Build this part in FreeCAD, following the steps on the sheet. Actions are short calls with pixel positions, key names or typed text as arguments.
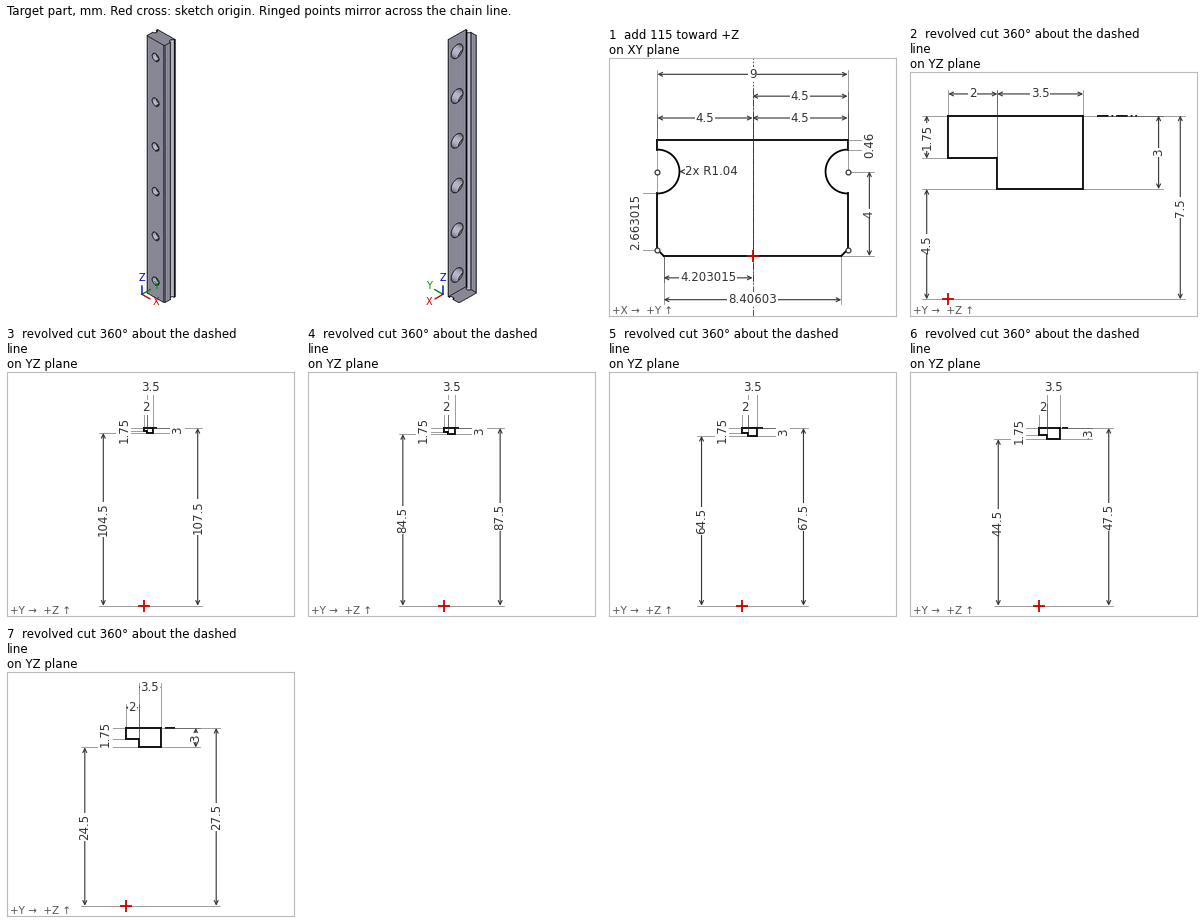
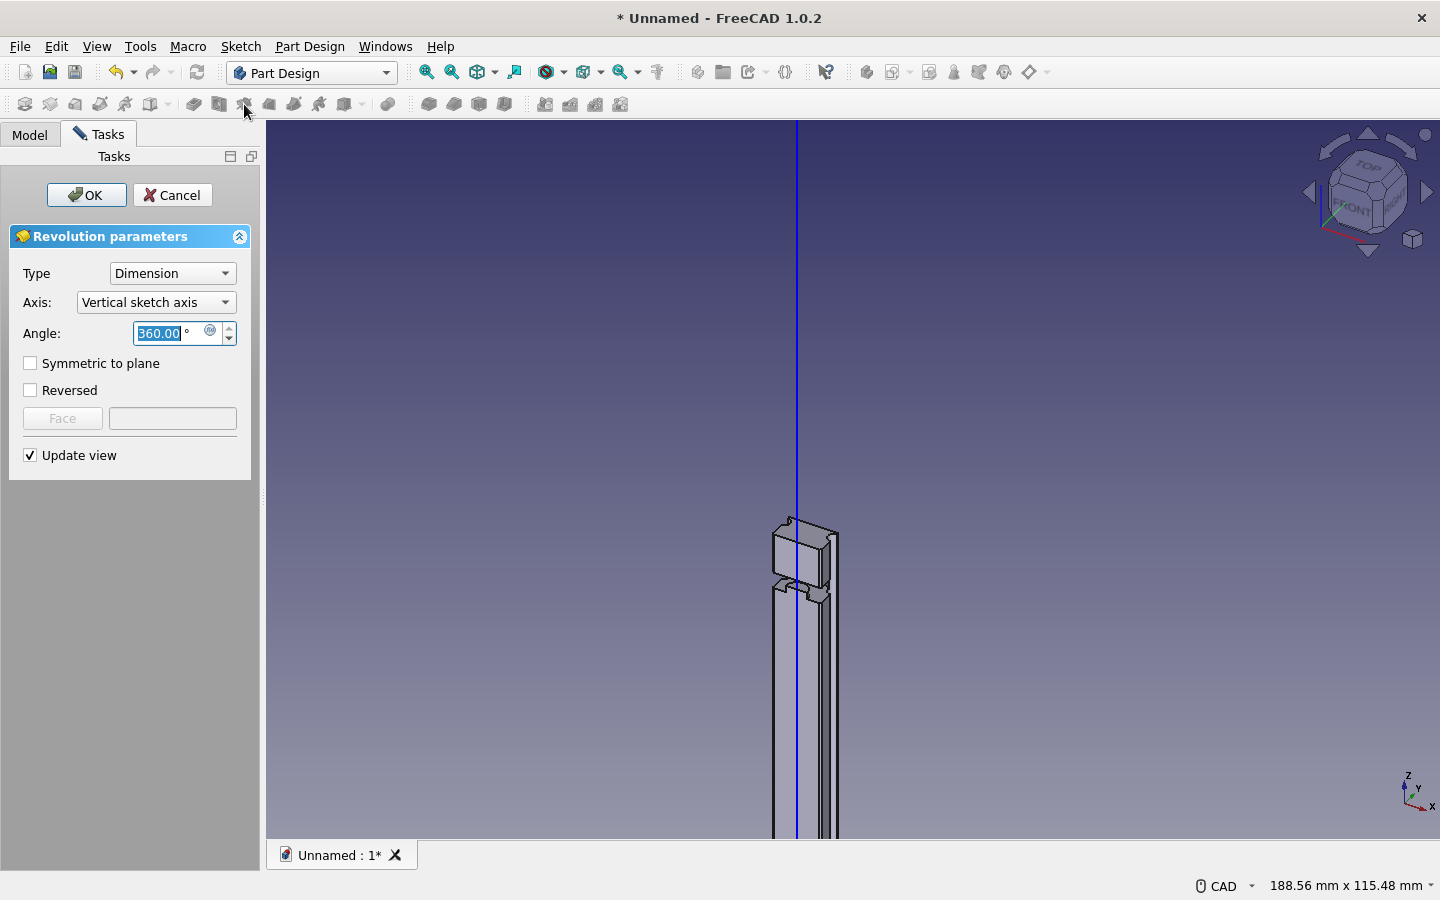
click(157, 302)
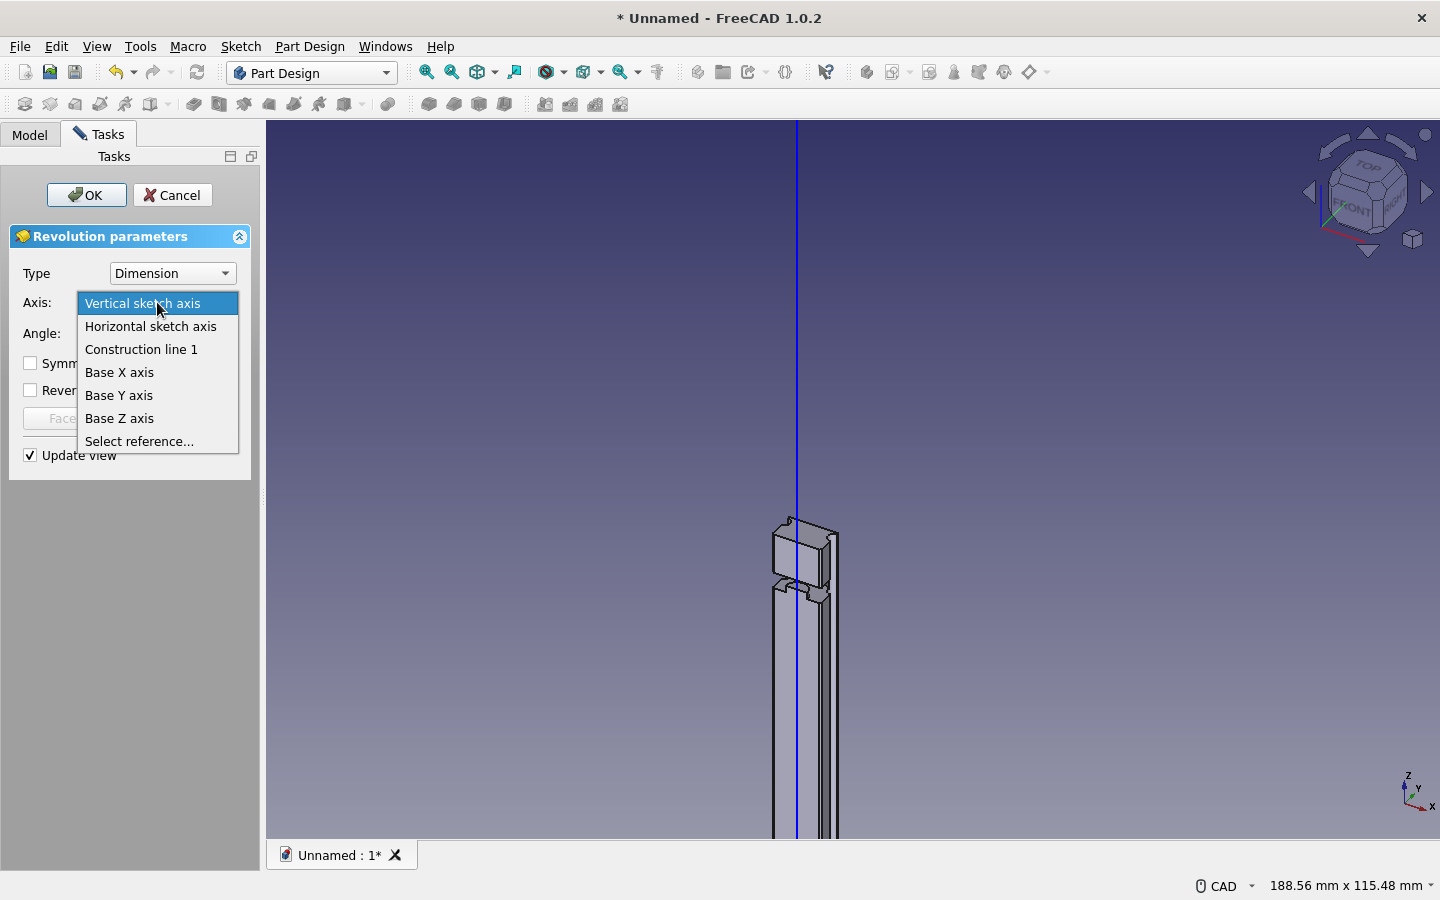
click(156, 350)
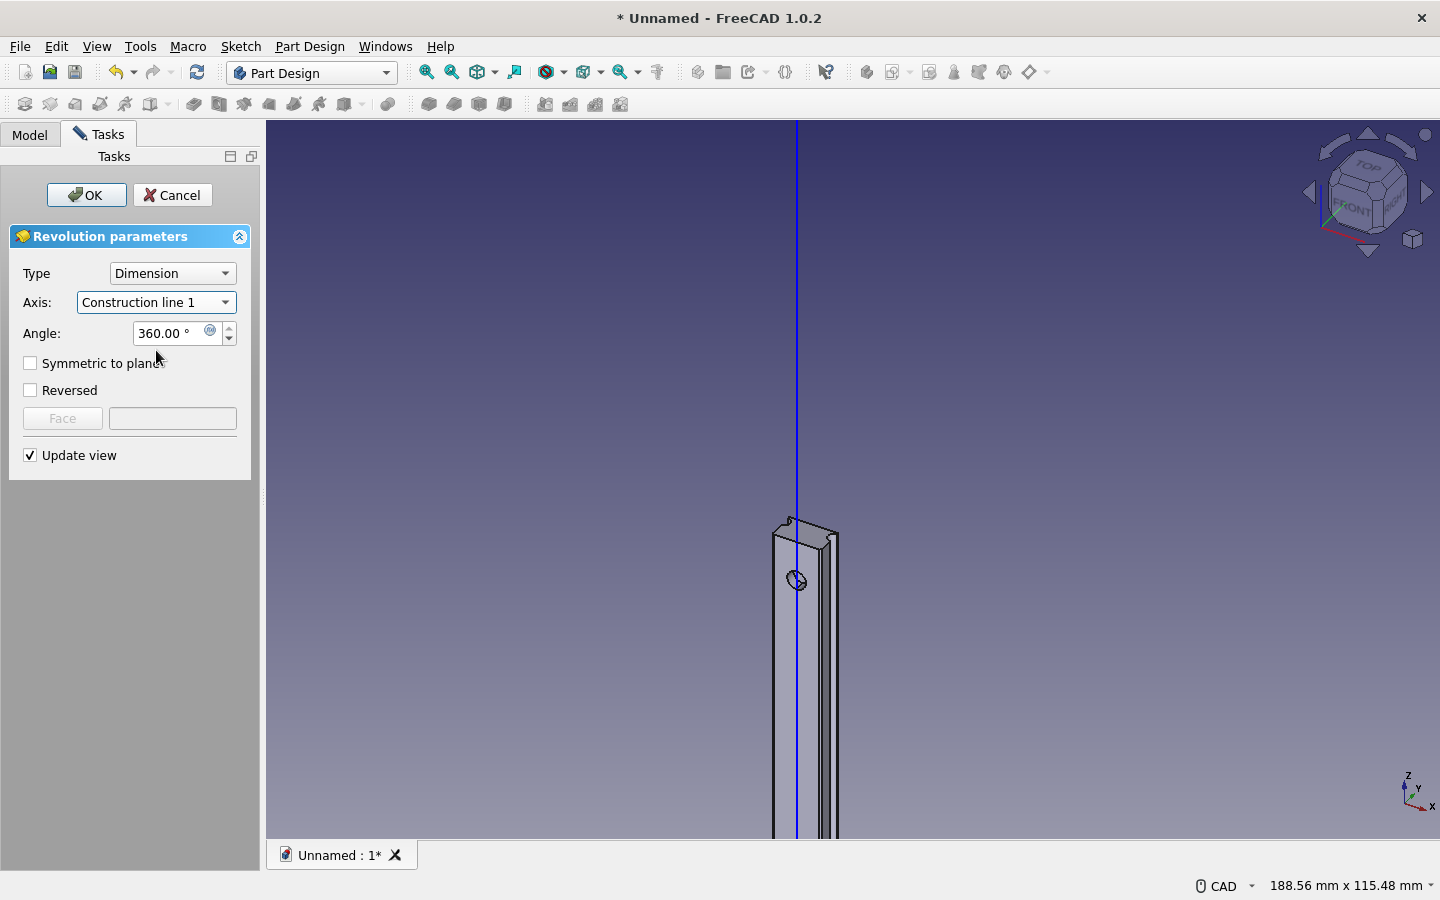
click(87, 195)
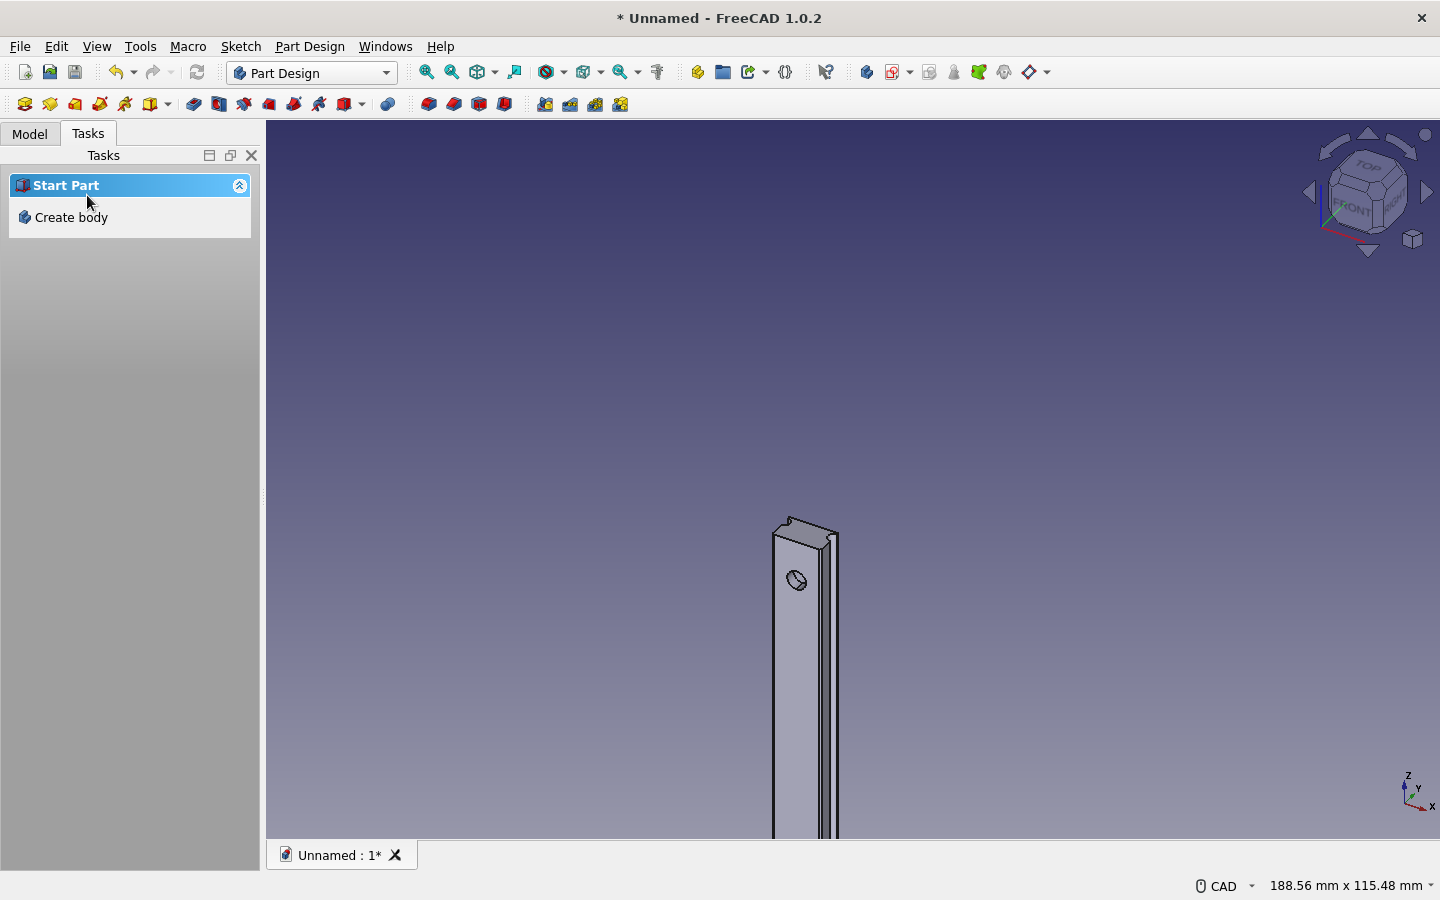
key(v)
key(f)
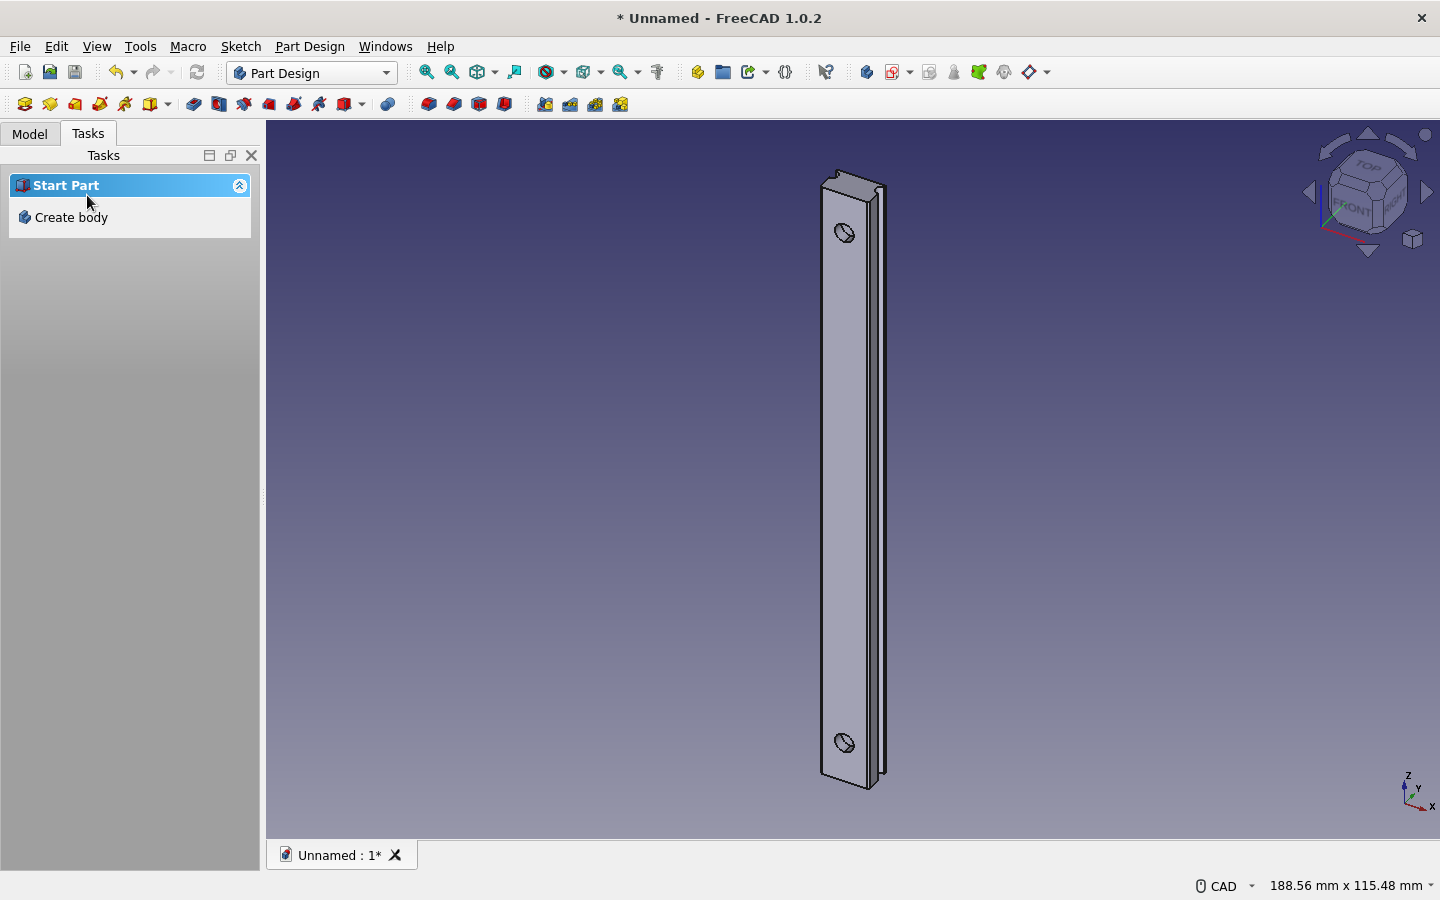
click(892, 72)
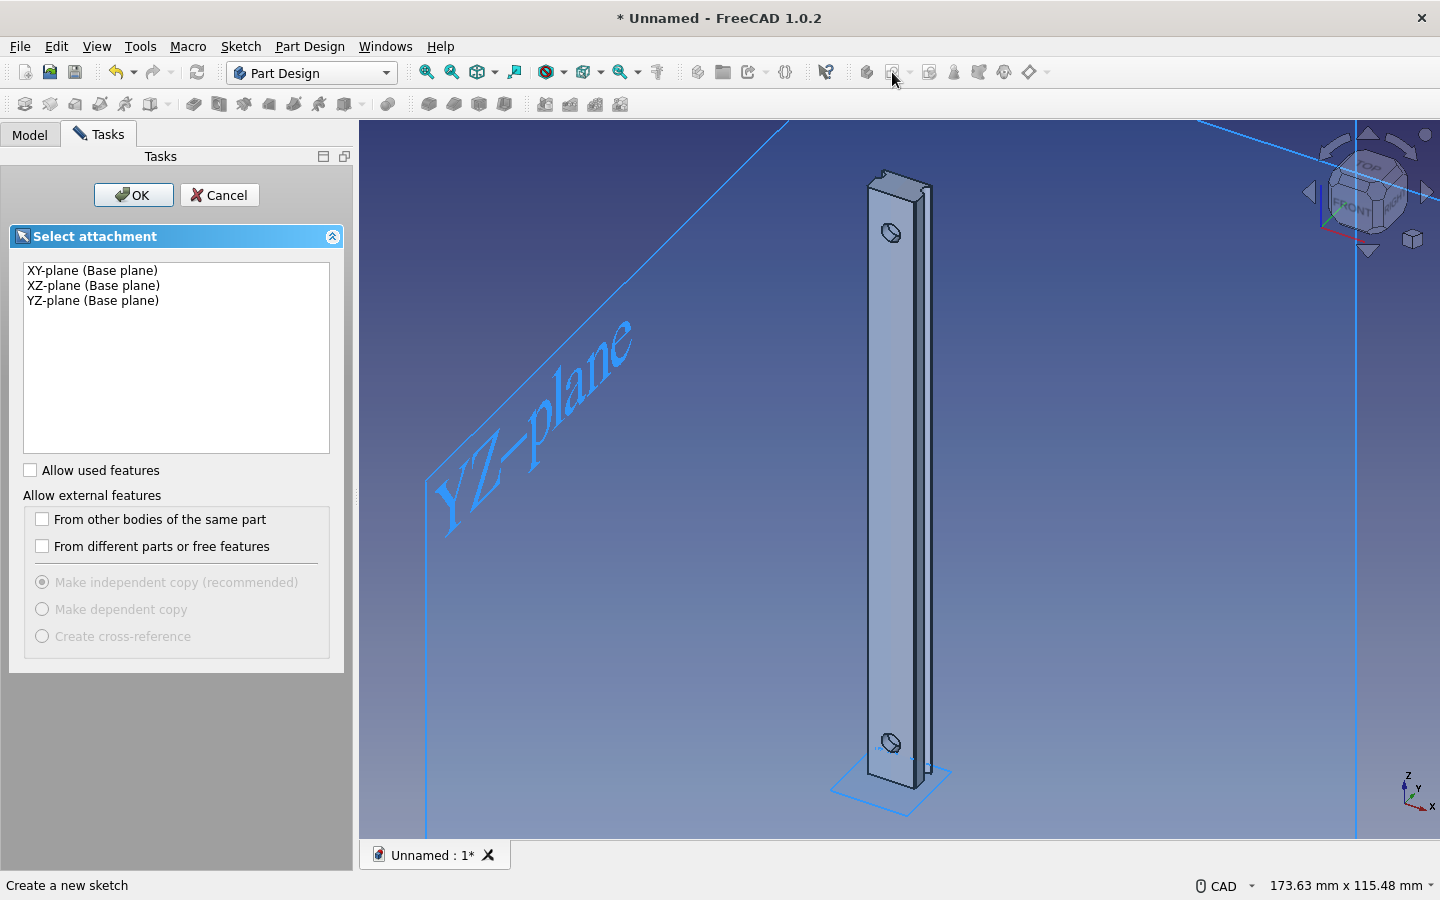
click(84, 300)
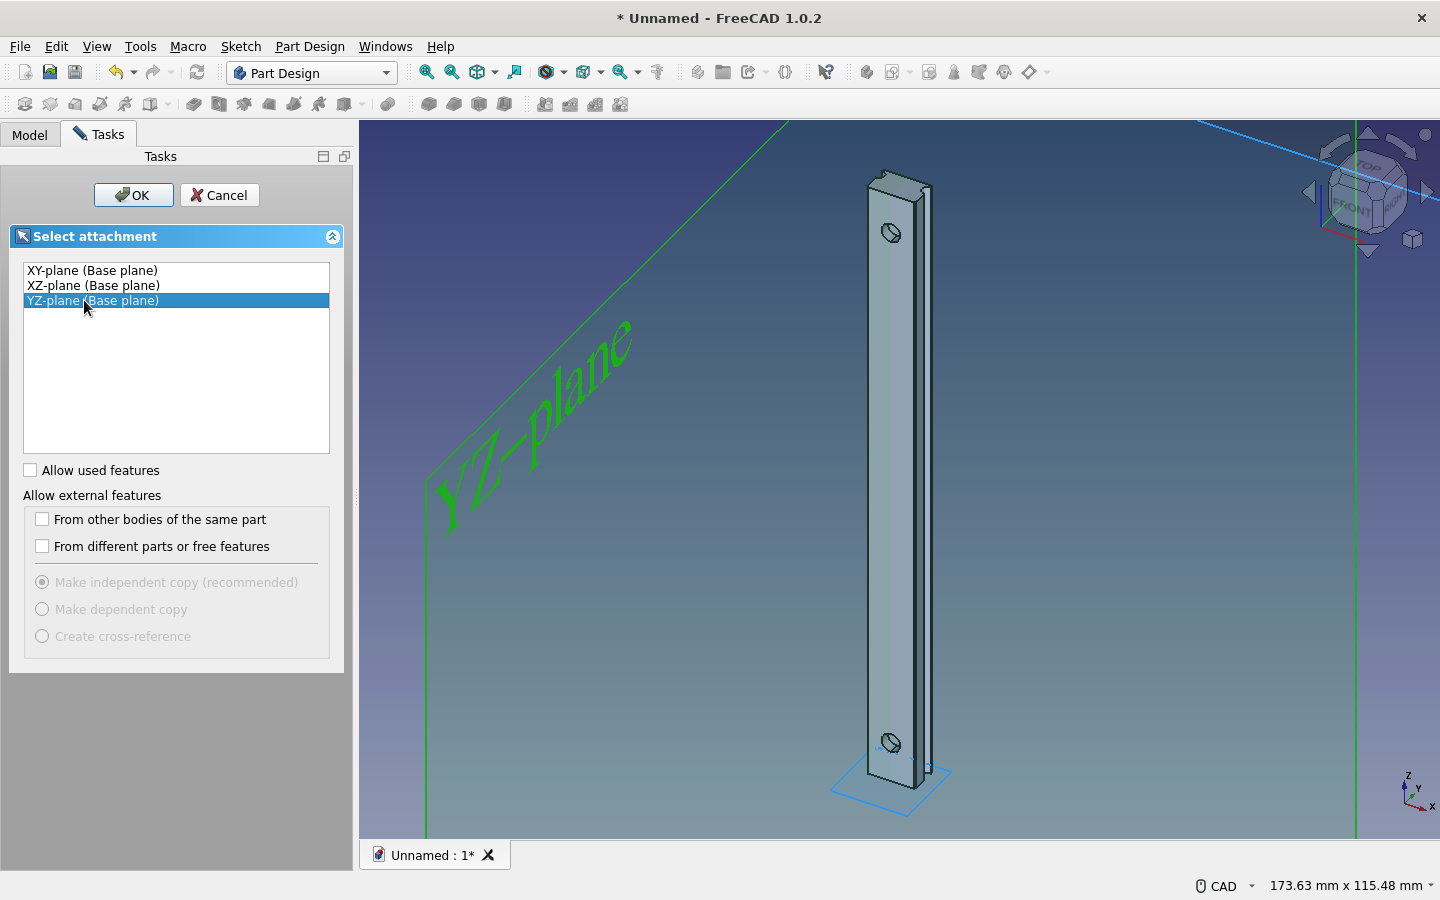
click(134, 195)